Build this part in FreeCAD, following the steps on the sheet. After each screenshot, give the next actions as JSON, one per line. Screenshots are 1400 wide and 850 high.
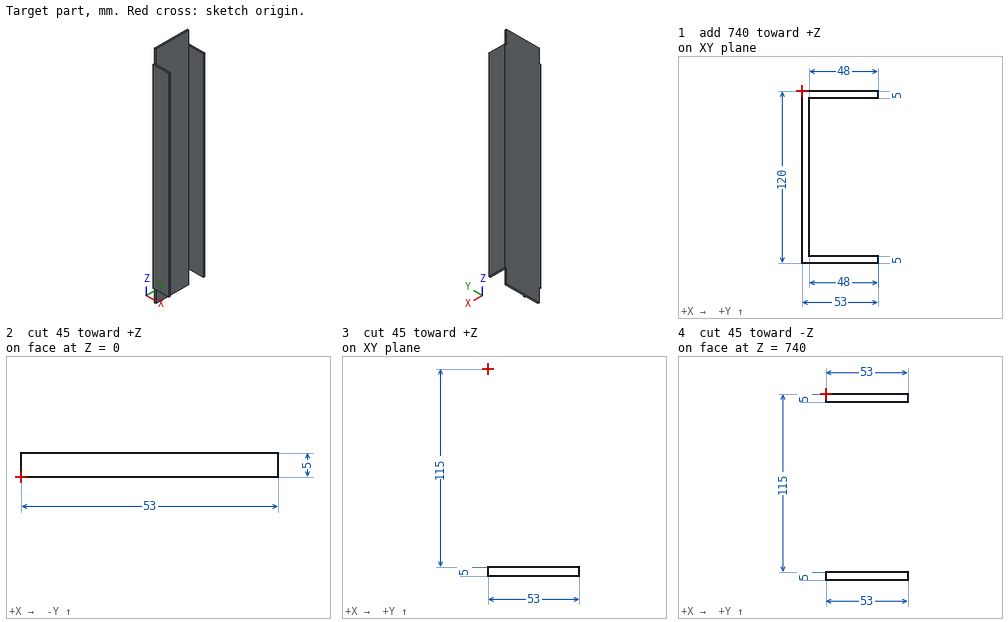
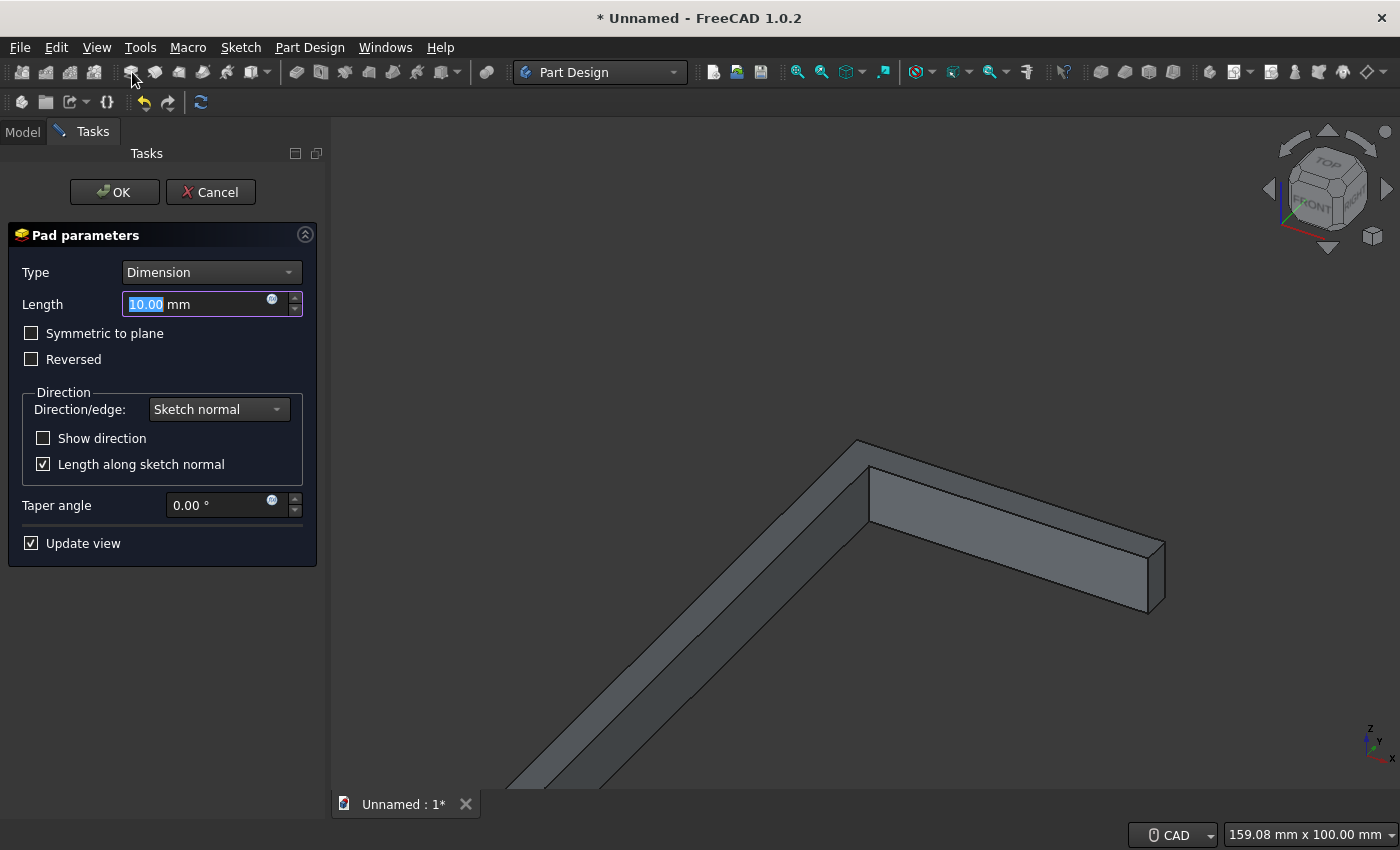
{"action": "type", "text": "740"}
{"action": "key", "text": "Tab"}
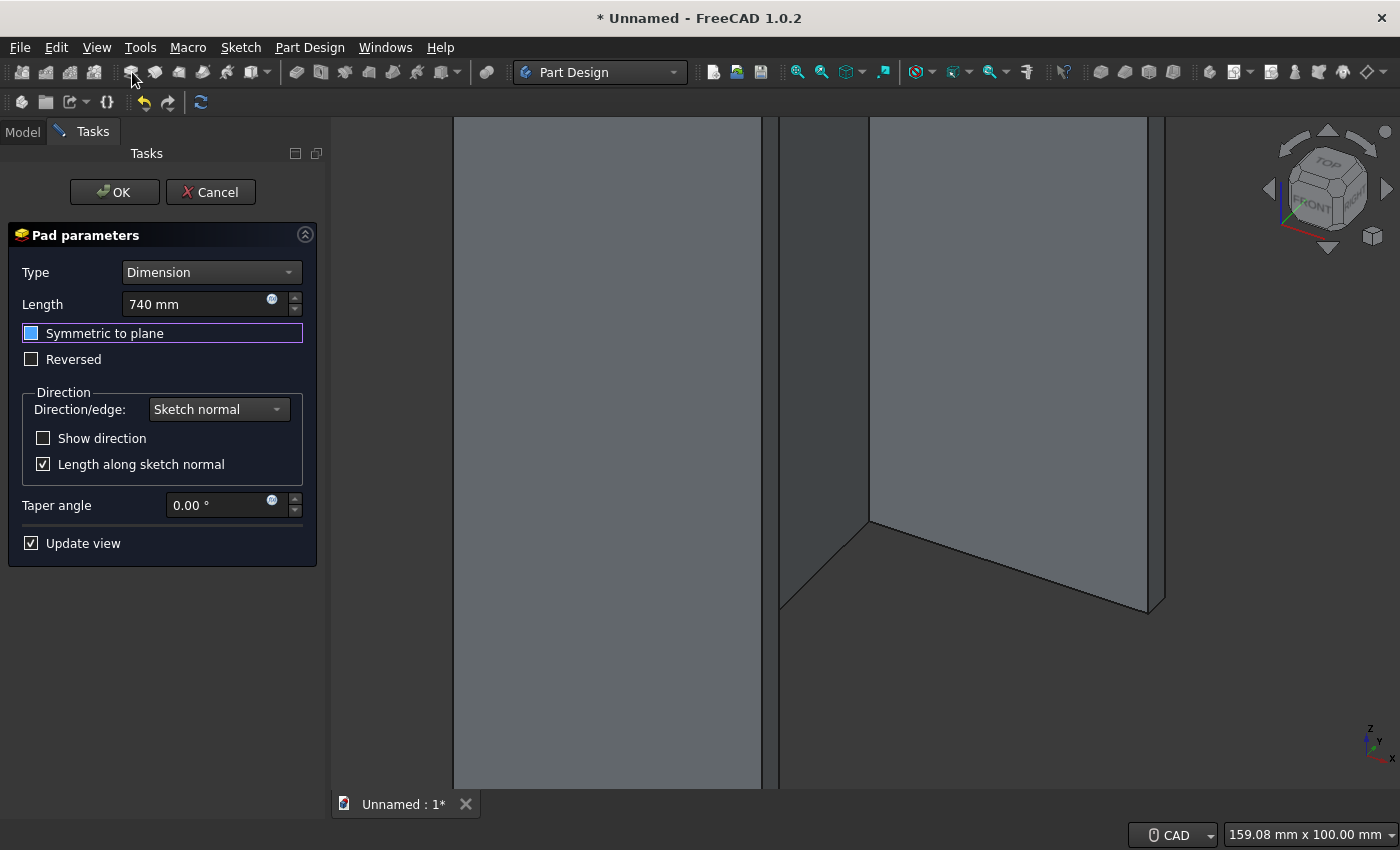
{"action": "left_click", "coordinate": [115, 192]}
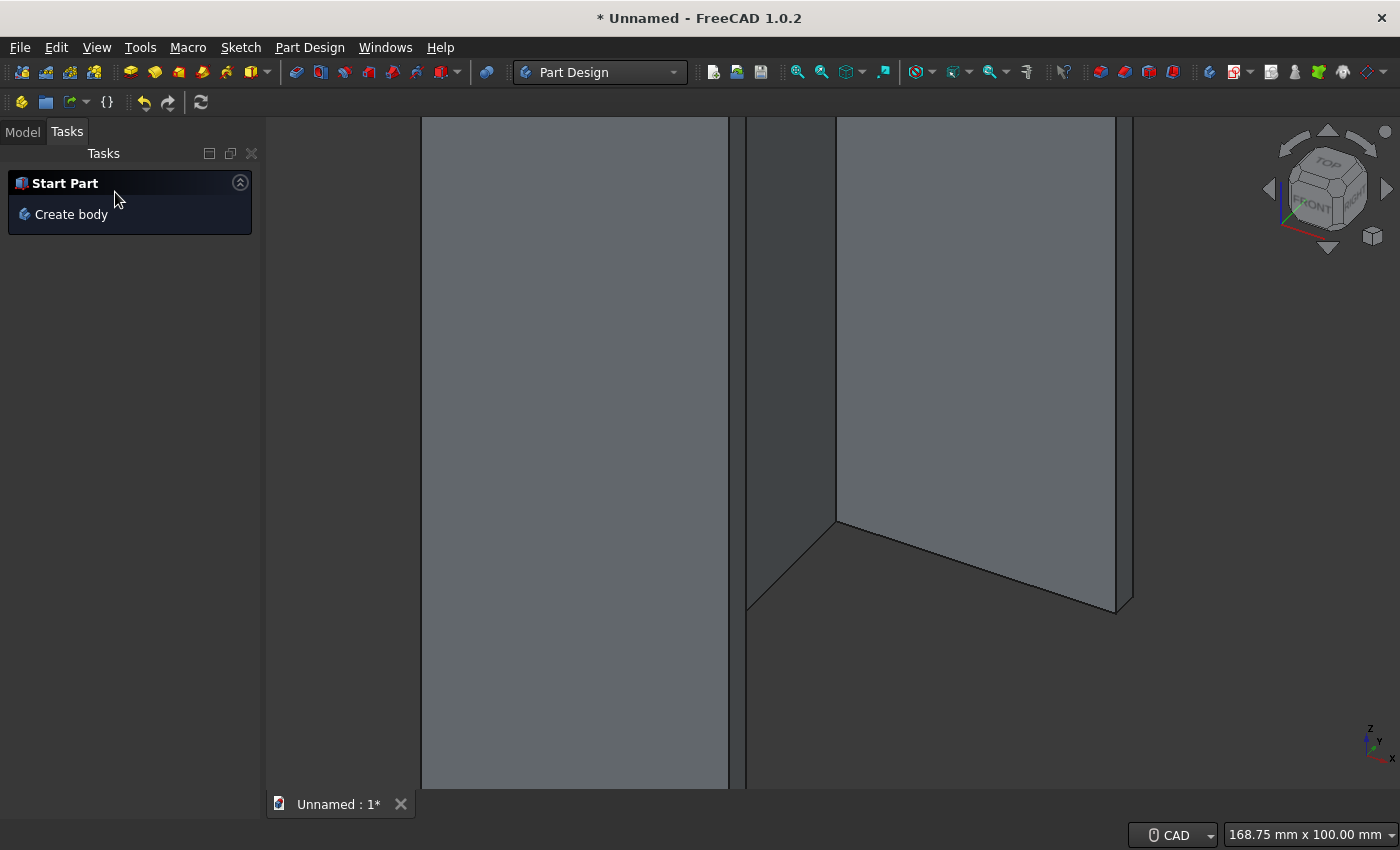
{"action": "left_click", "coordinate": [798, 72]}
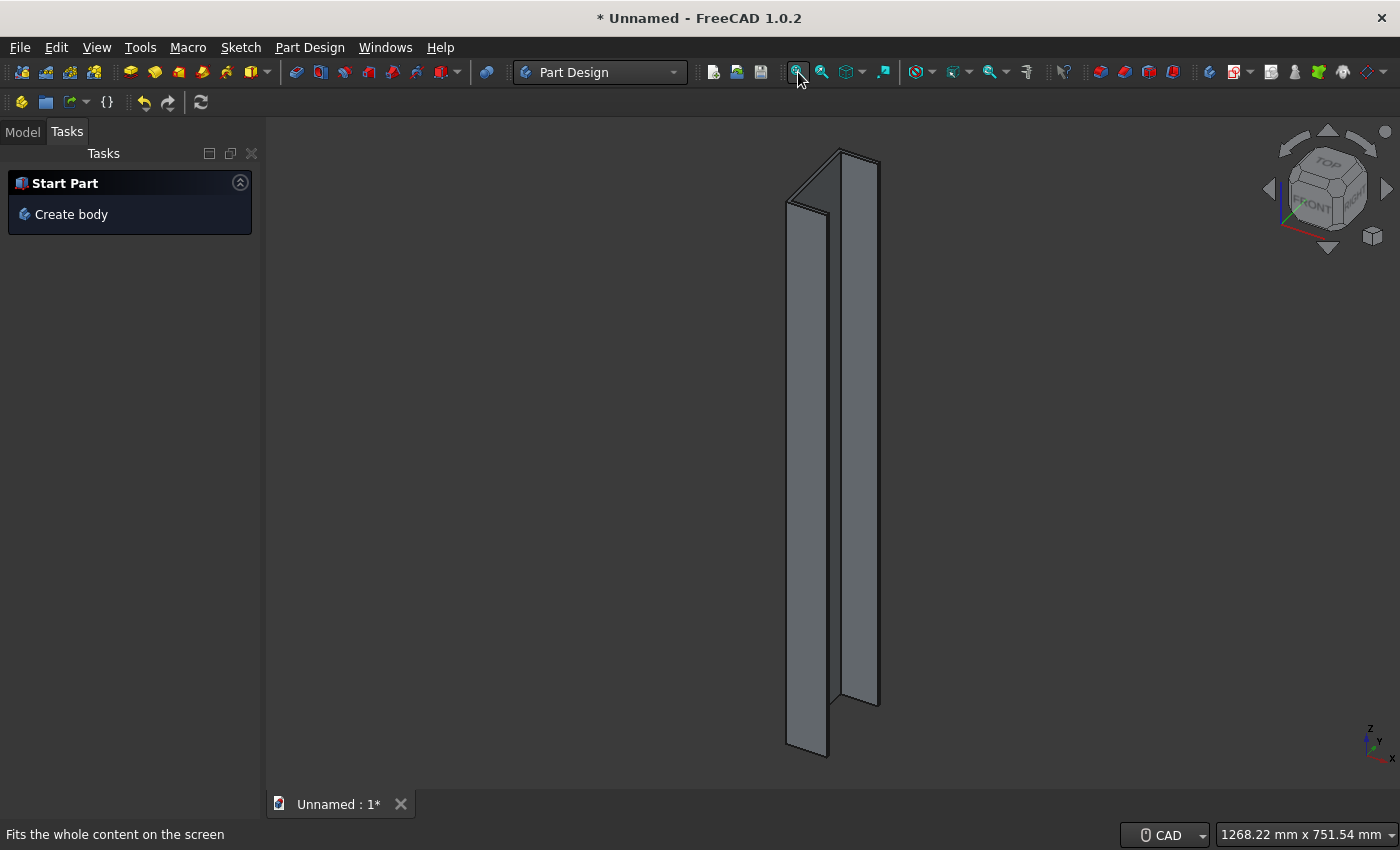
{"action": "key", "text": "5"}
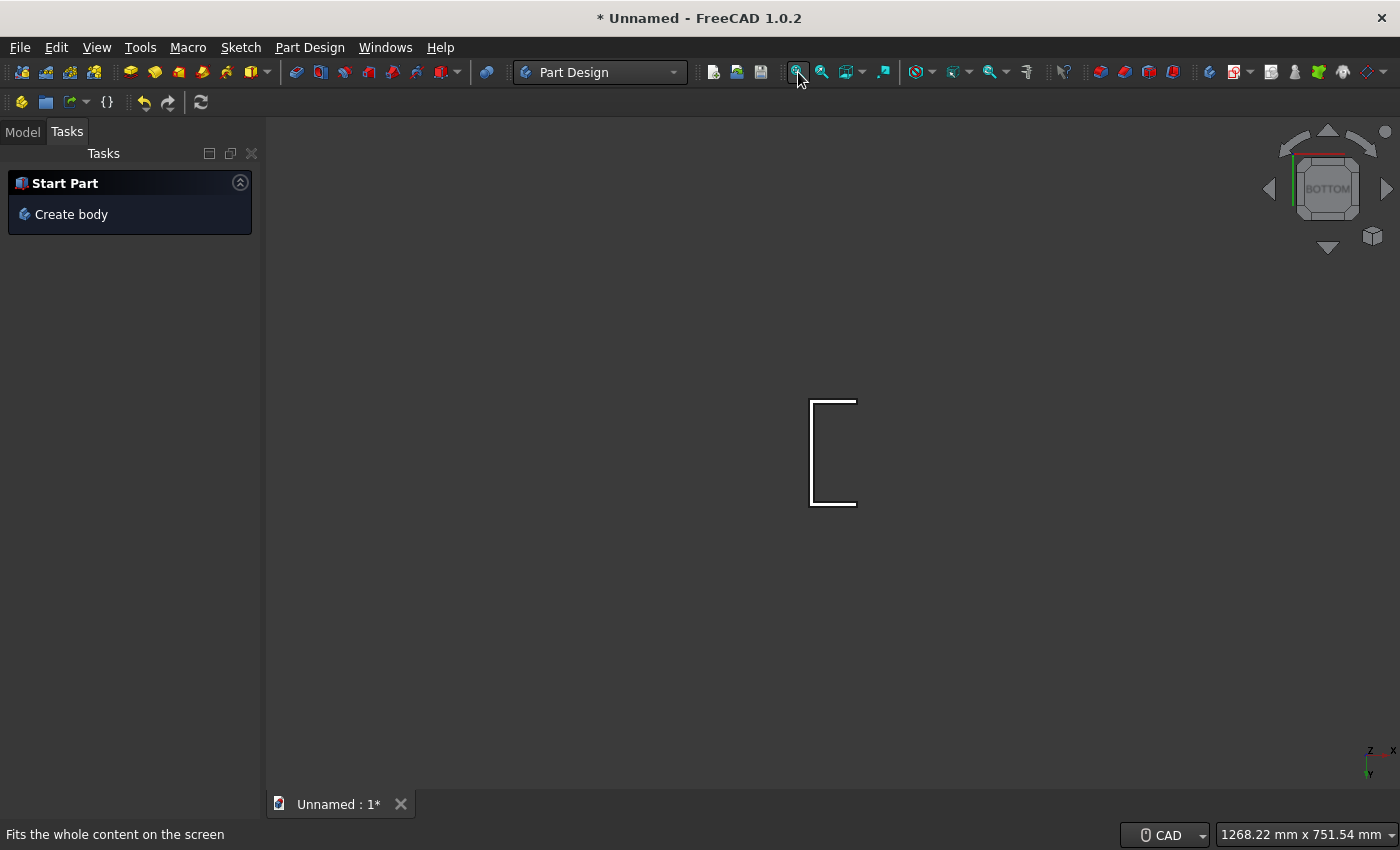
{"action": "left_click", "coordinate": [798, 72]}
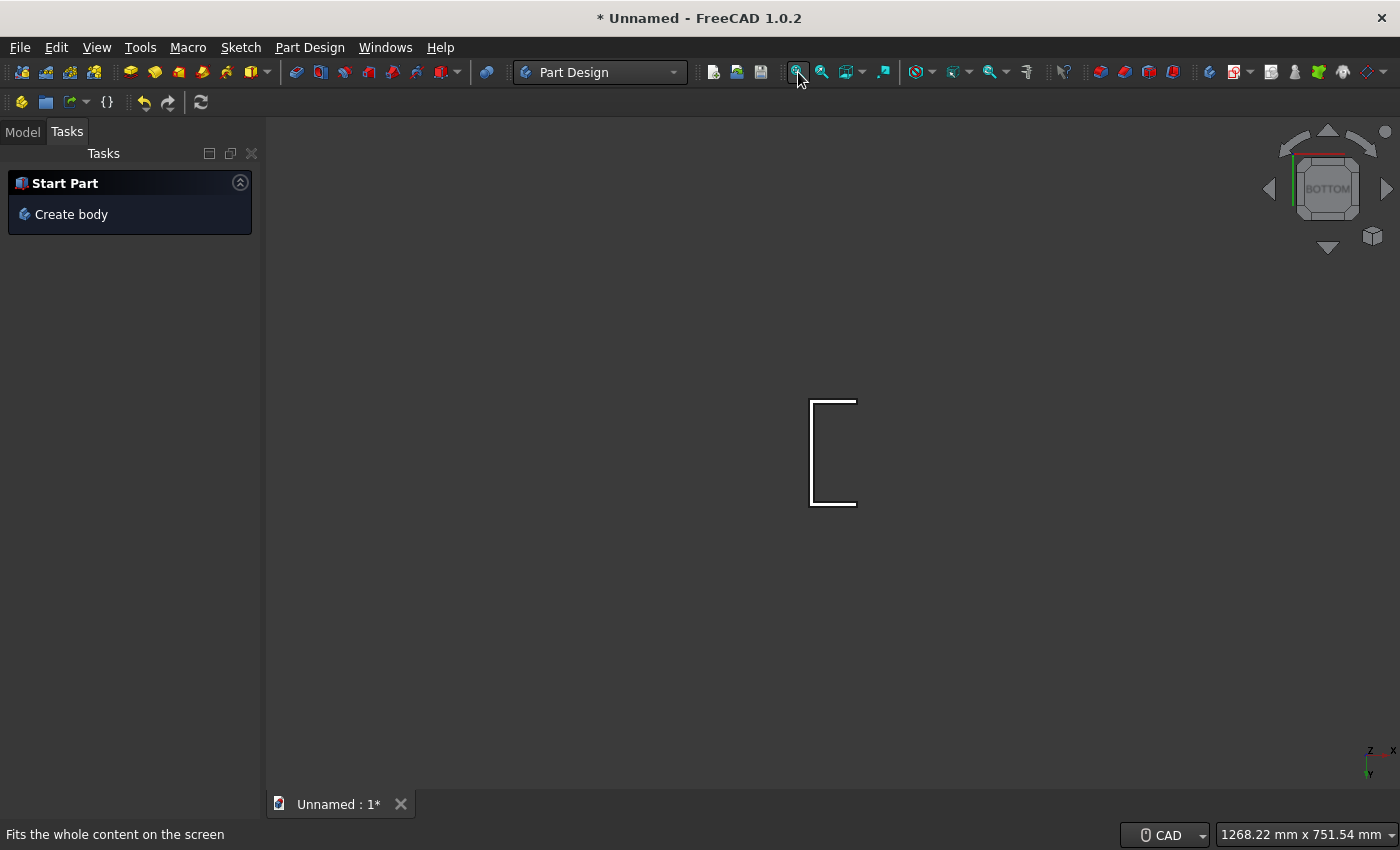
{"action": "scroll", "coordinate": [813, 498], "scroll_direction": "up", "scroll_amount": 13}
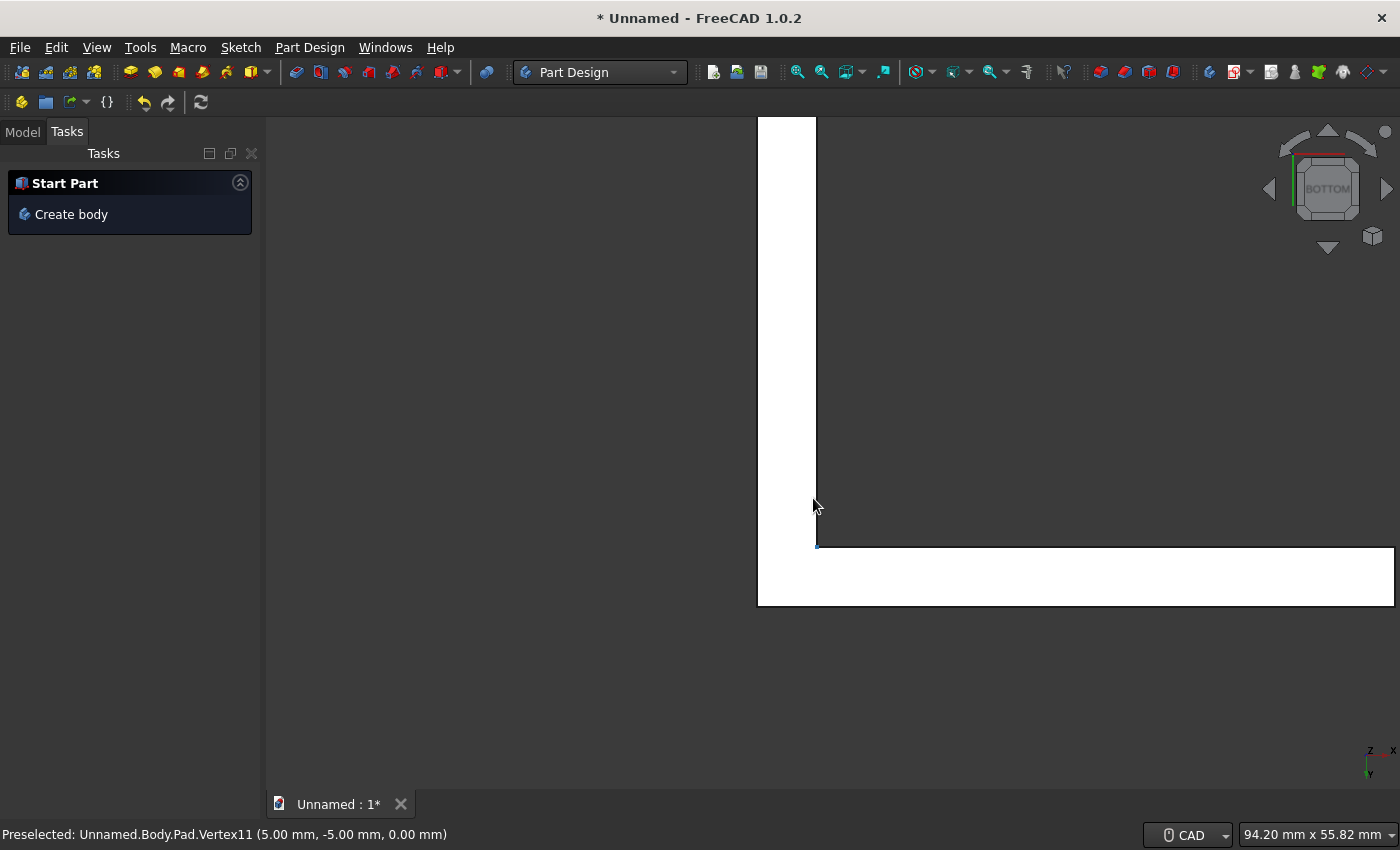
{"action": "left_click", "coordinate": [803, 503]}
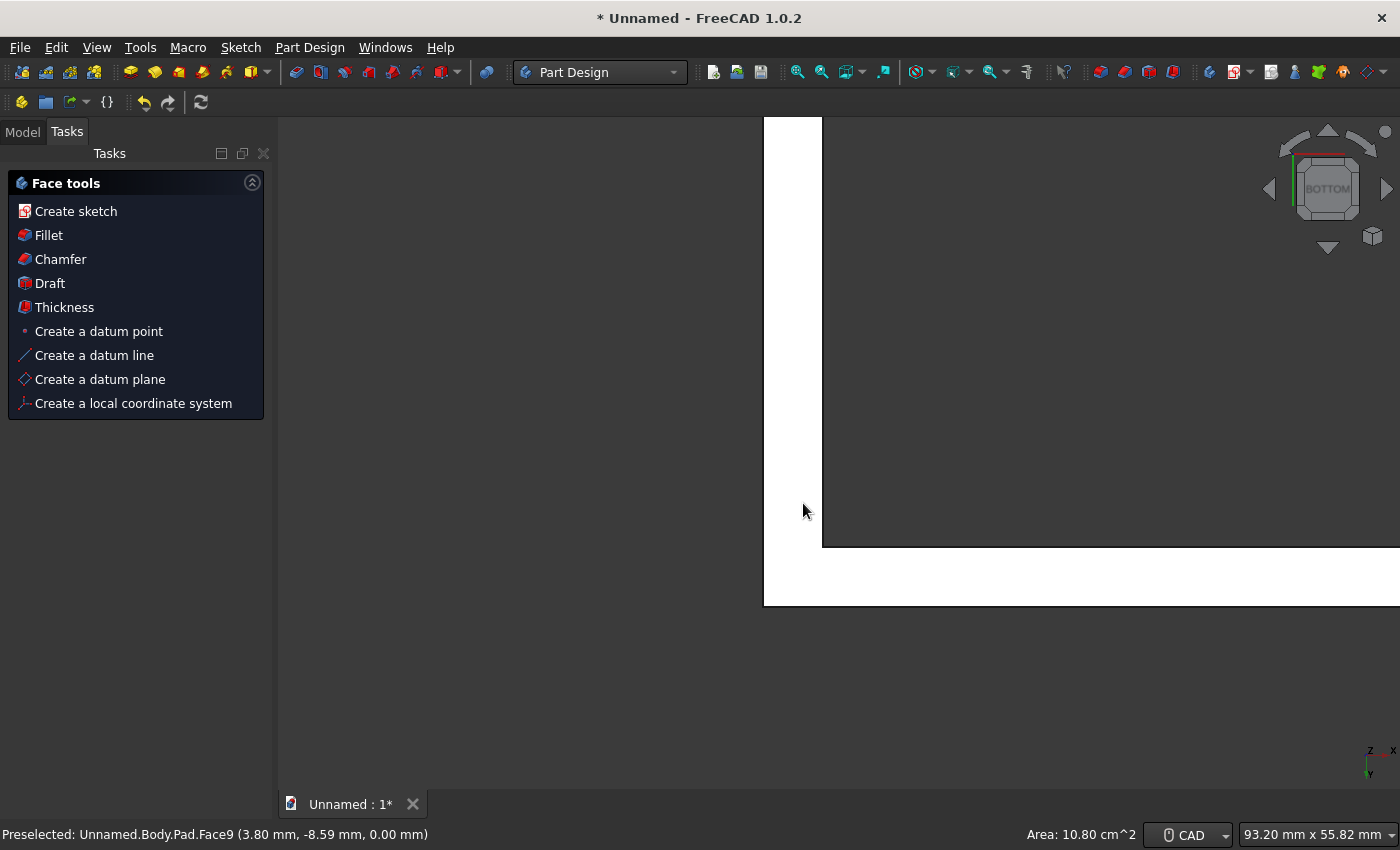
{"action": "left_click", "coordinate": [1234, 72]}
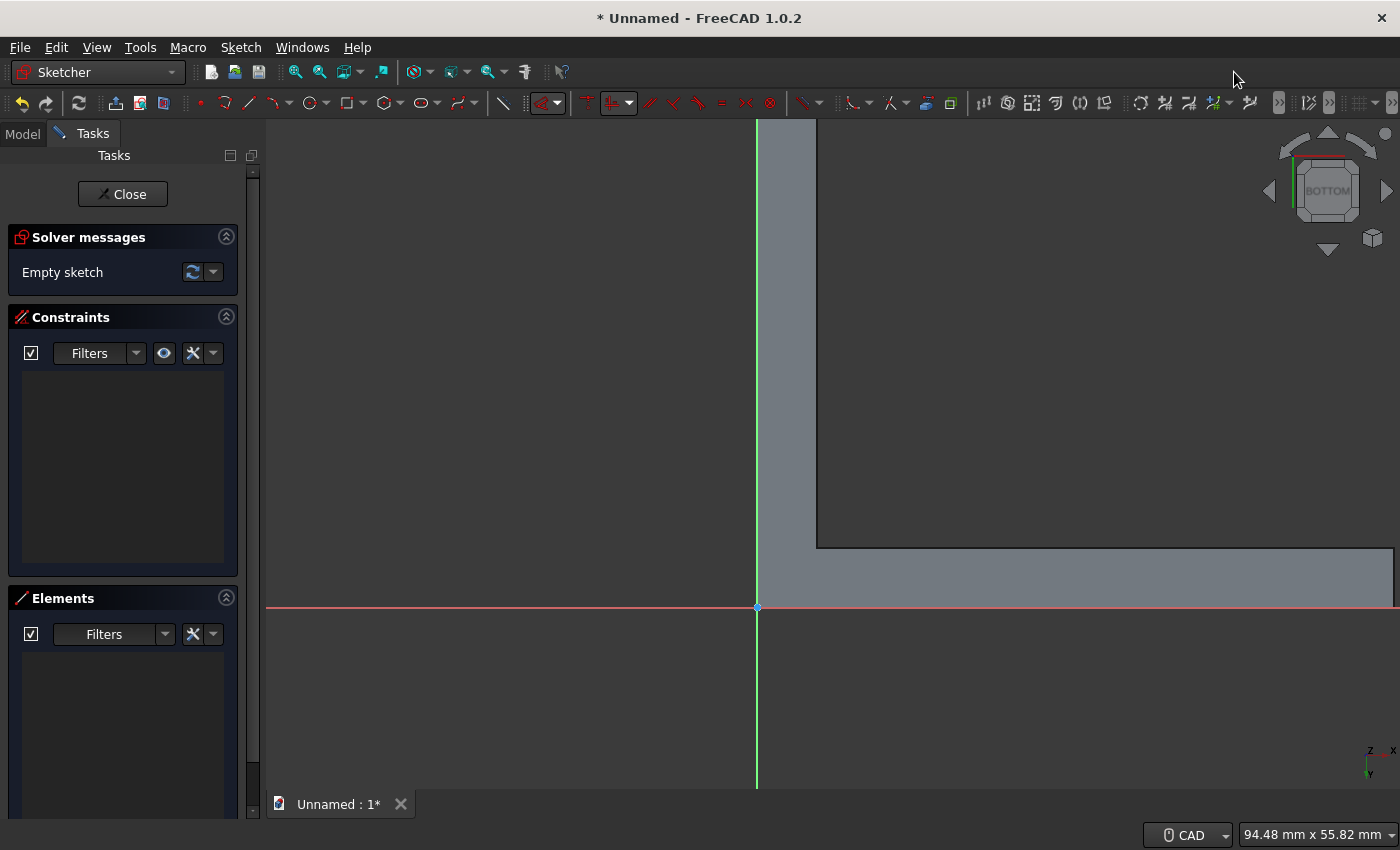
{"action": "scroll", "coordinate": [294, 147], "scroll_direction": "down", "scroll_amount": 1}